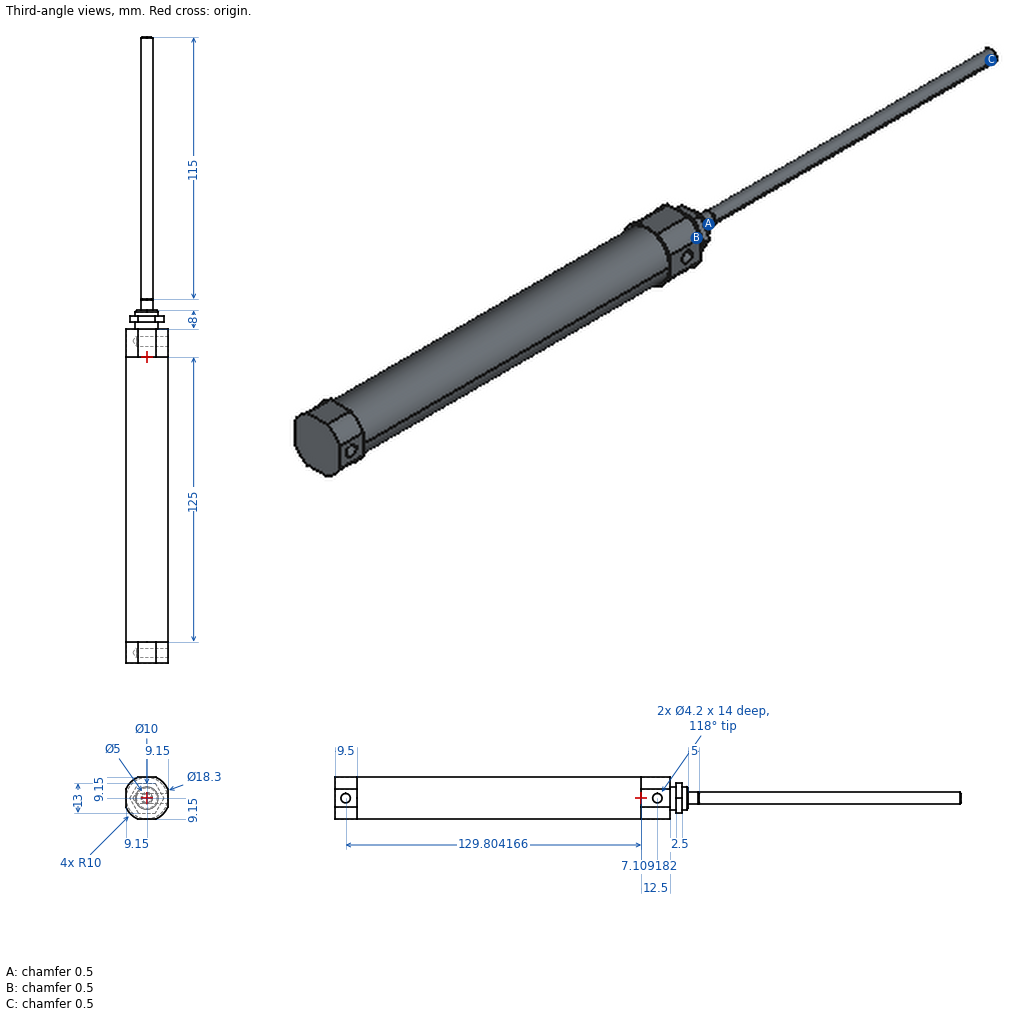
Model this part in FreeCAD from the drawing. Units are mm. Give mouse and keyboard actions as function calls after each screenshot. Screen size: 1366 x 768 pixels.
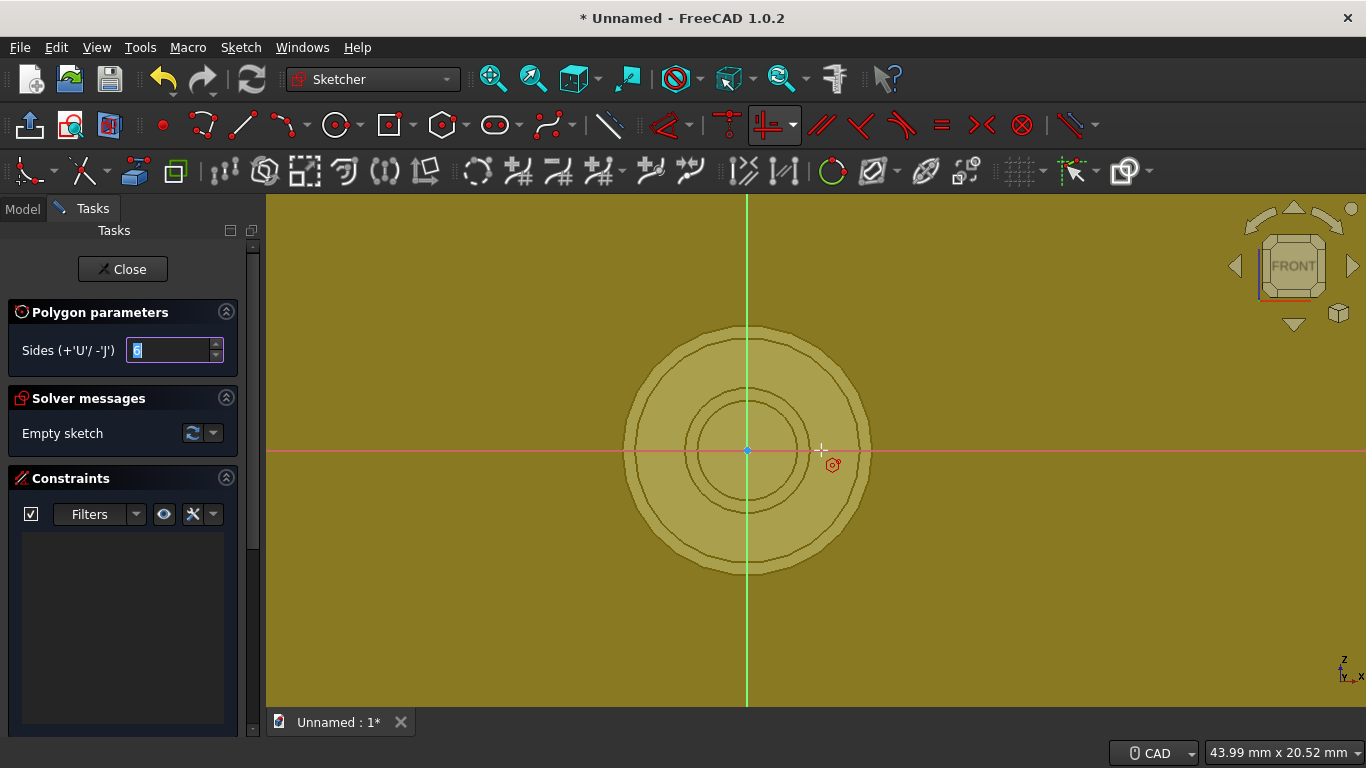
click(747, 451)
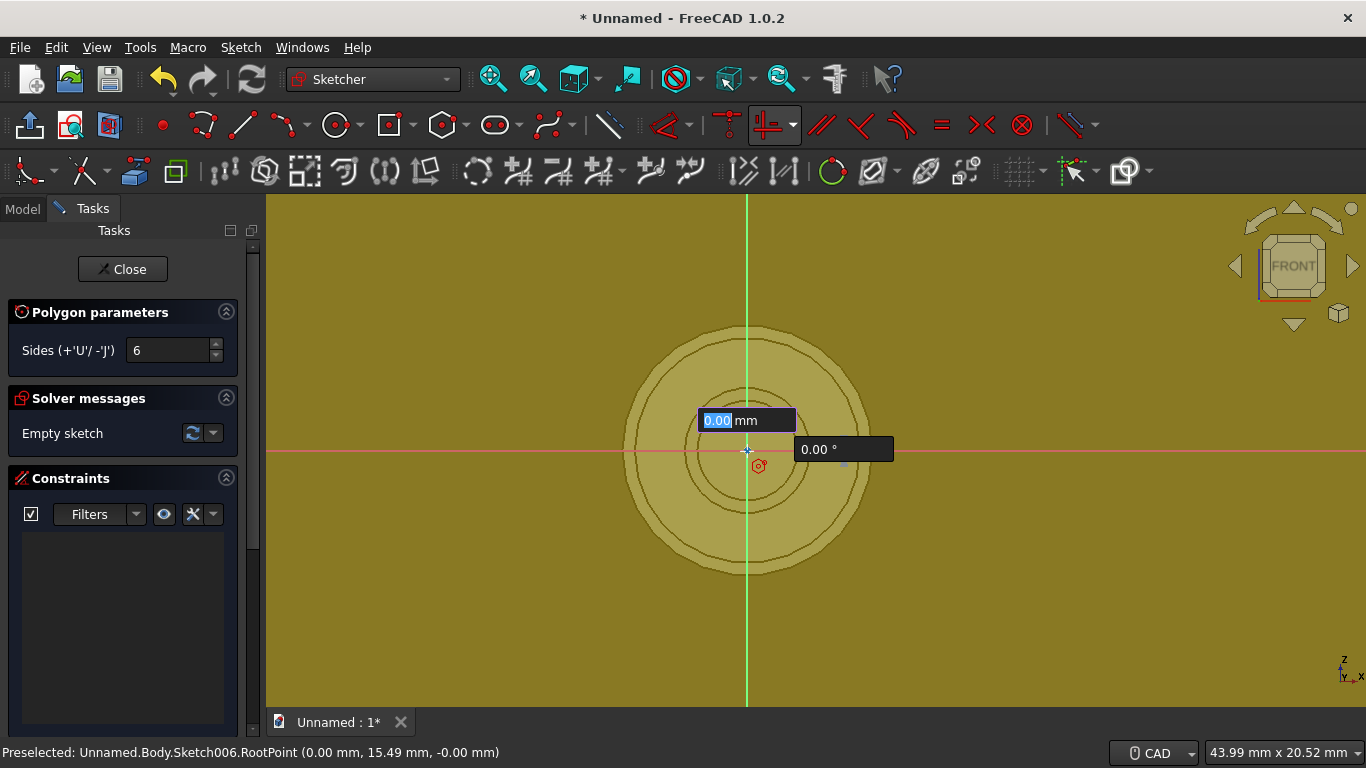
click(935, 451)
key(Escape)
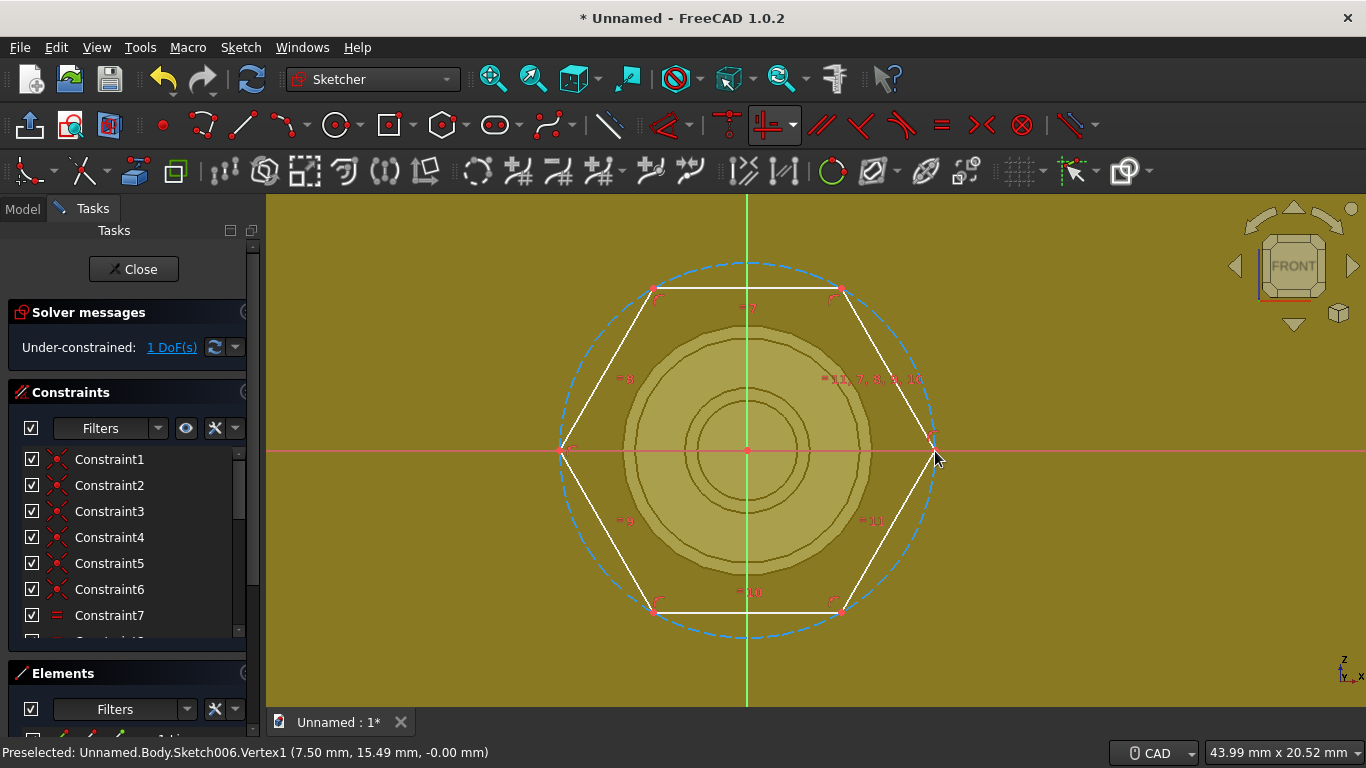
key(d)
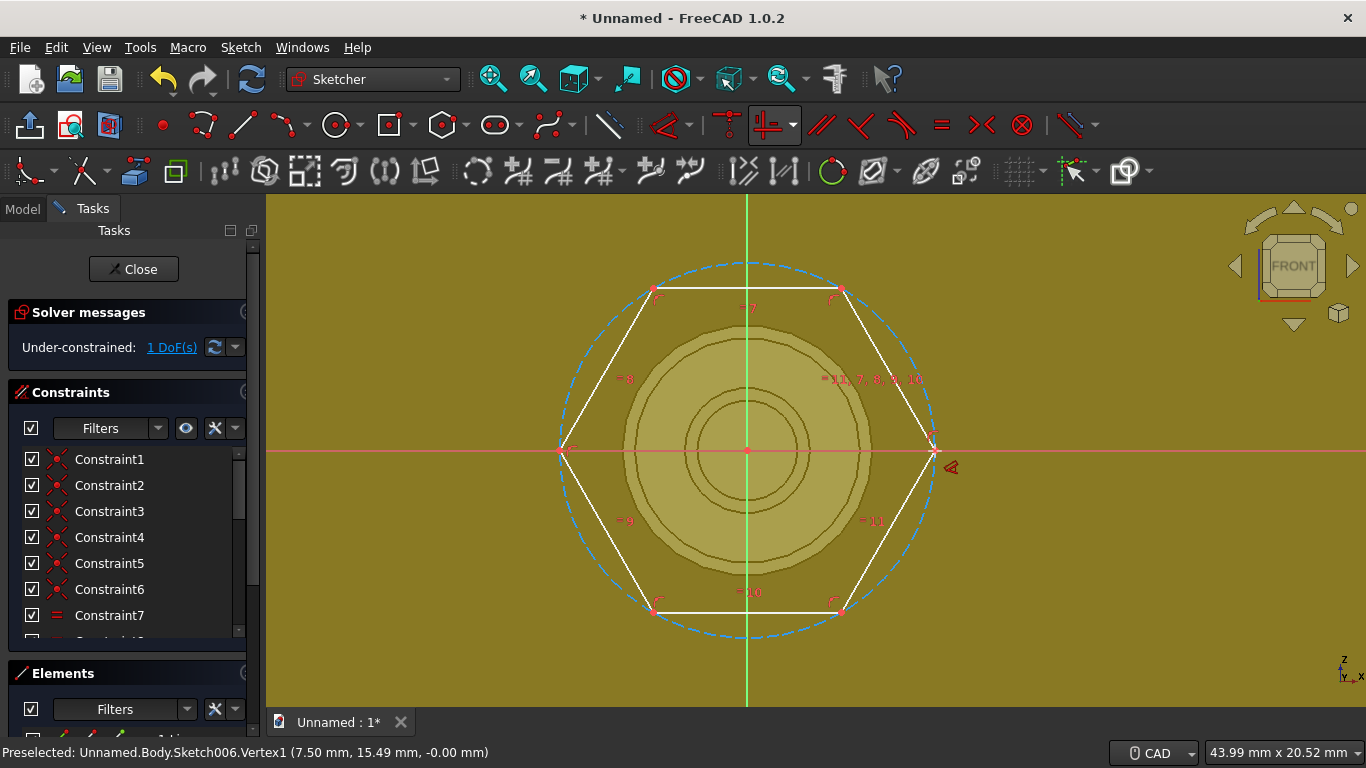
click(654, 613)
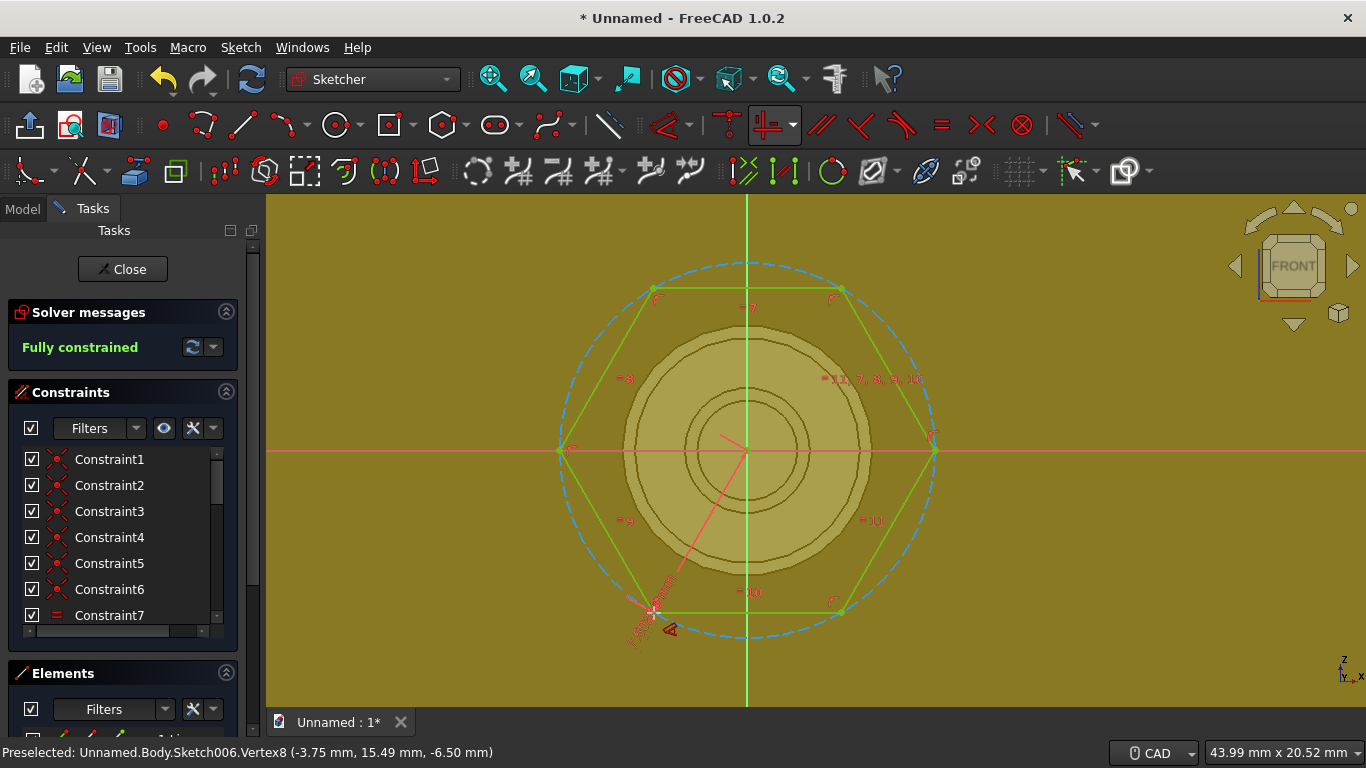
click(841, 288)
click(875, 376)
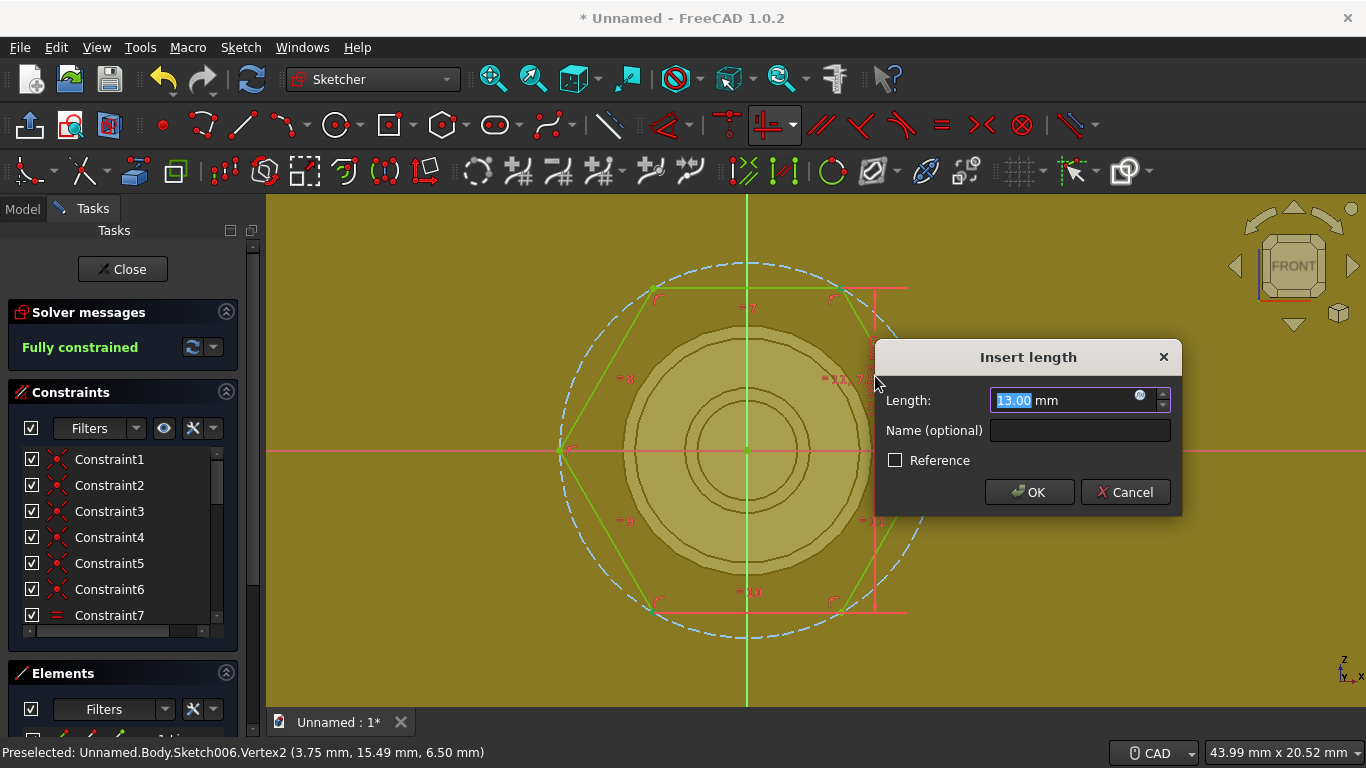
text(13)
key(Return)
key(Escape)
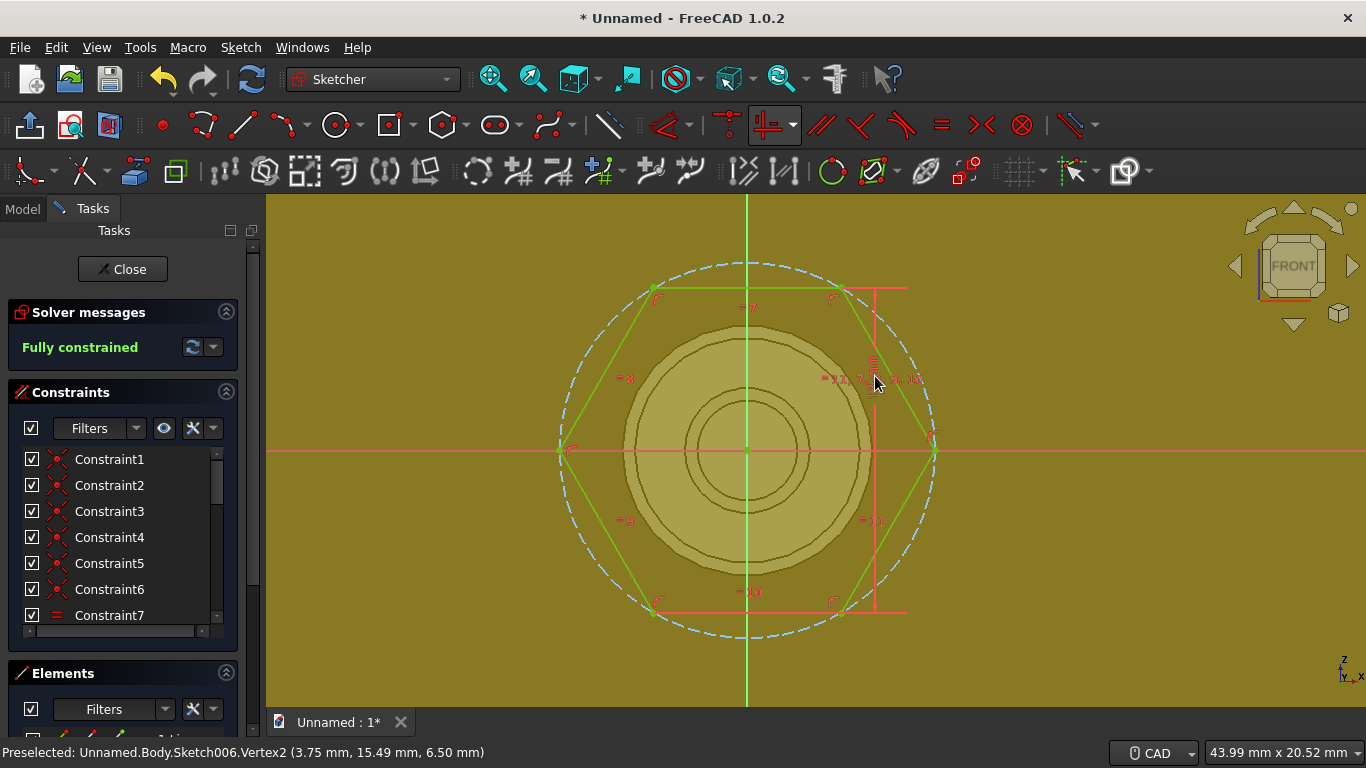
click(123, 269)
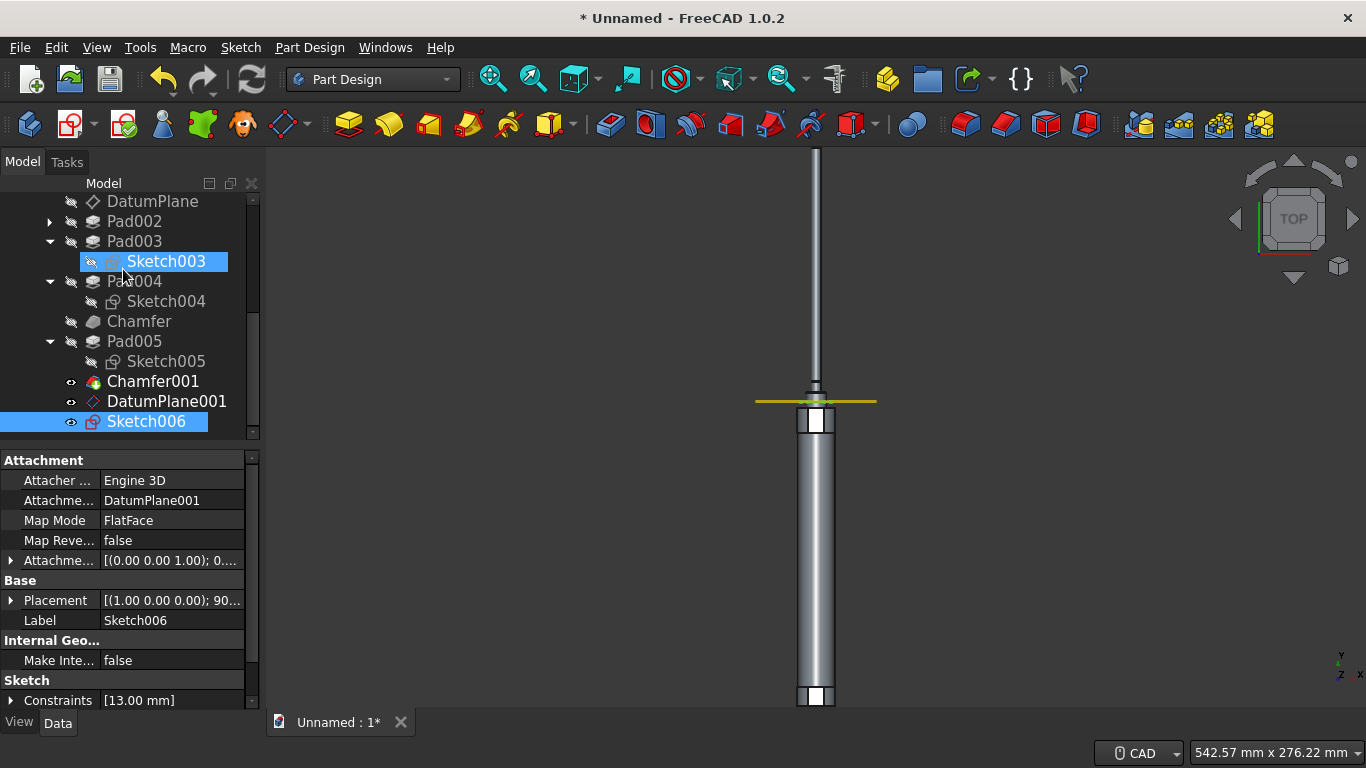
click(350, 124)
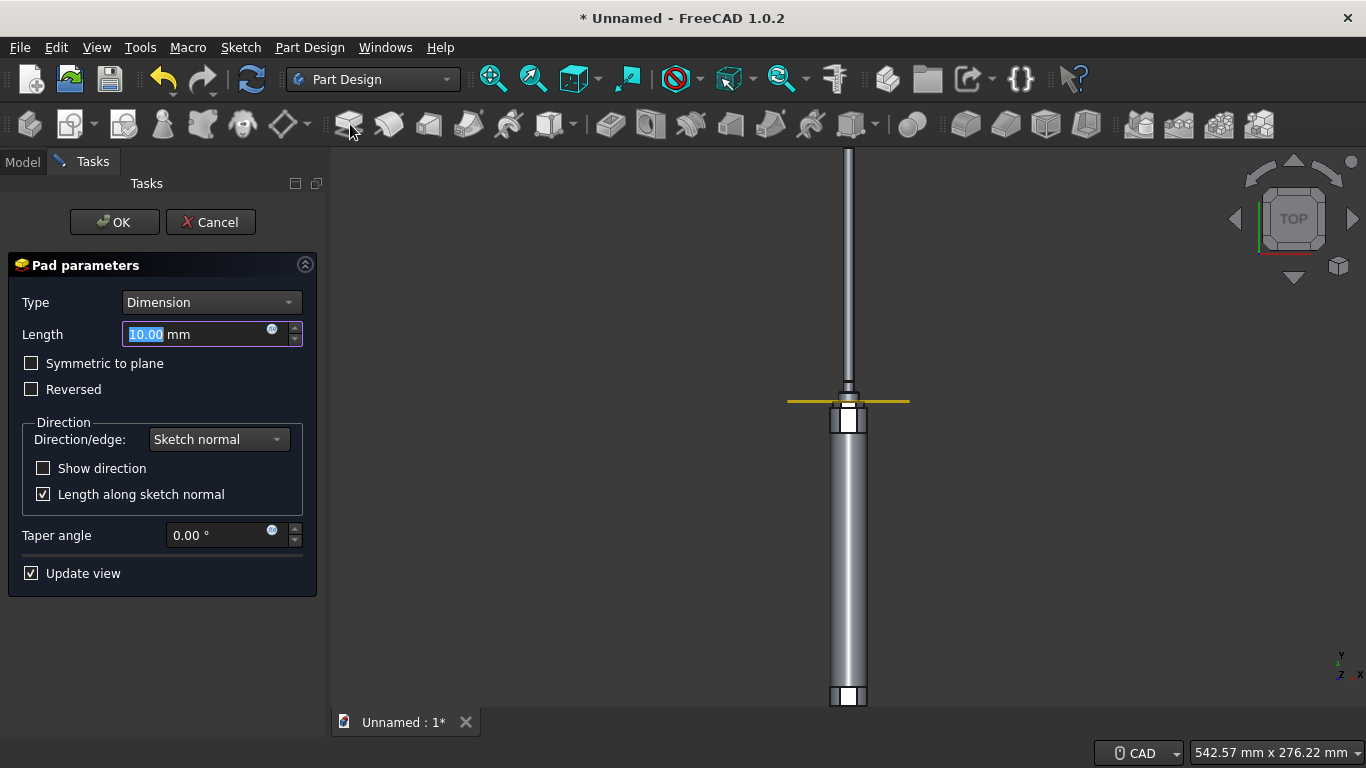
text(2.5)
key(Tab)